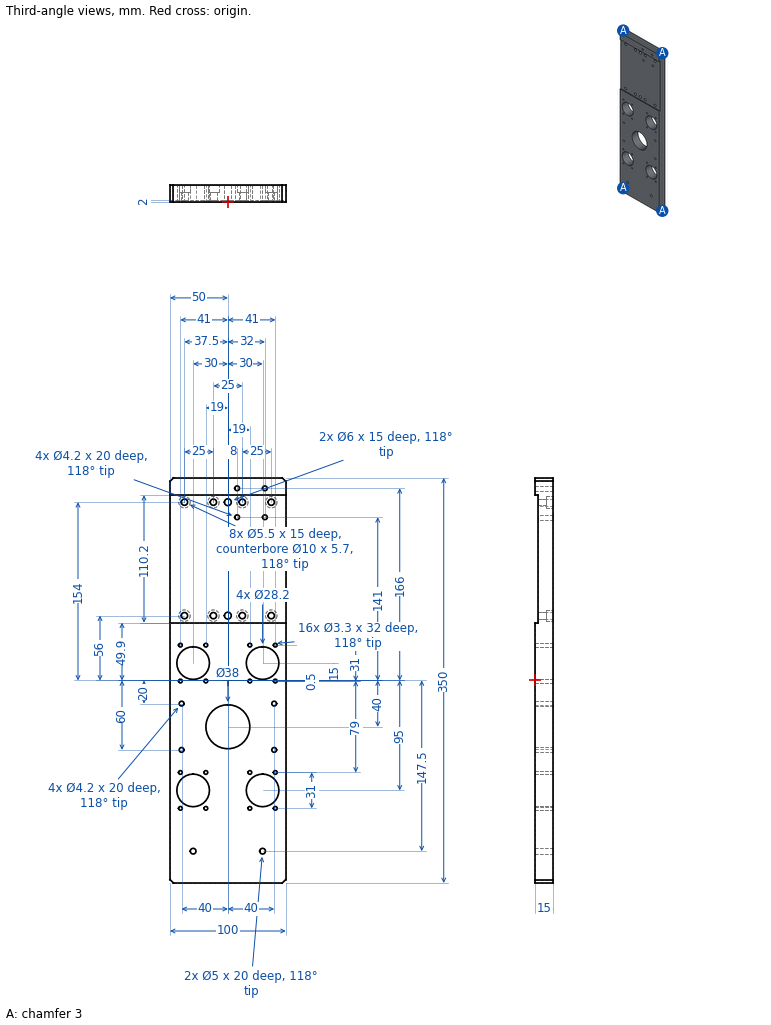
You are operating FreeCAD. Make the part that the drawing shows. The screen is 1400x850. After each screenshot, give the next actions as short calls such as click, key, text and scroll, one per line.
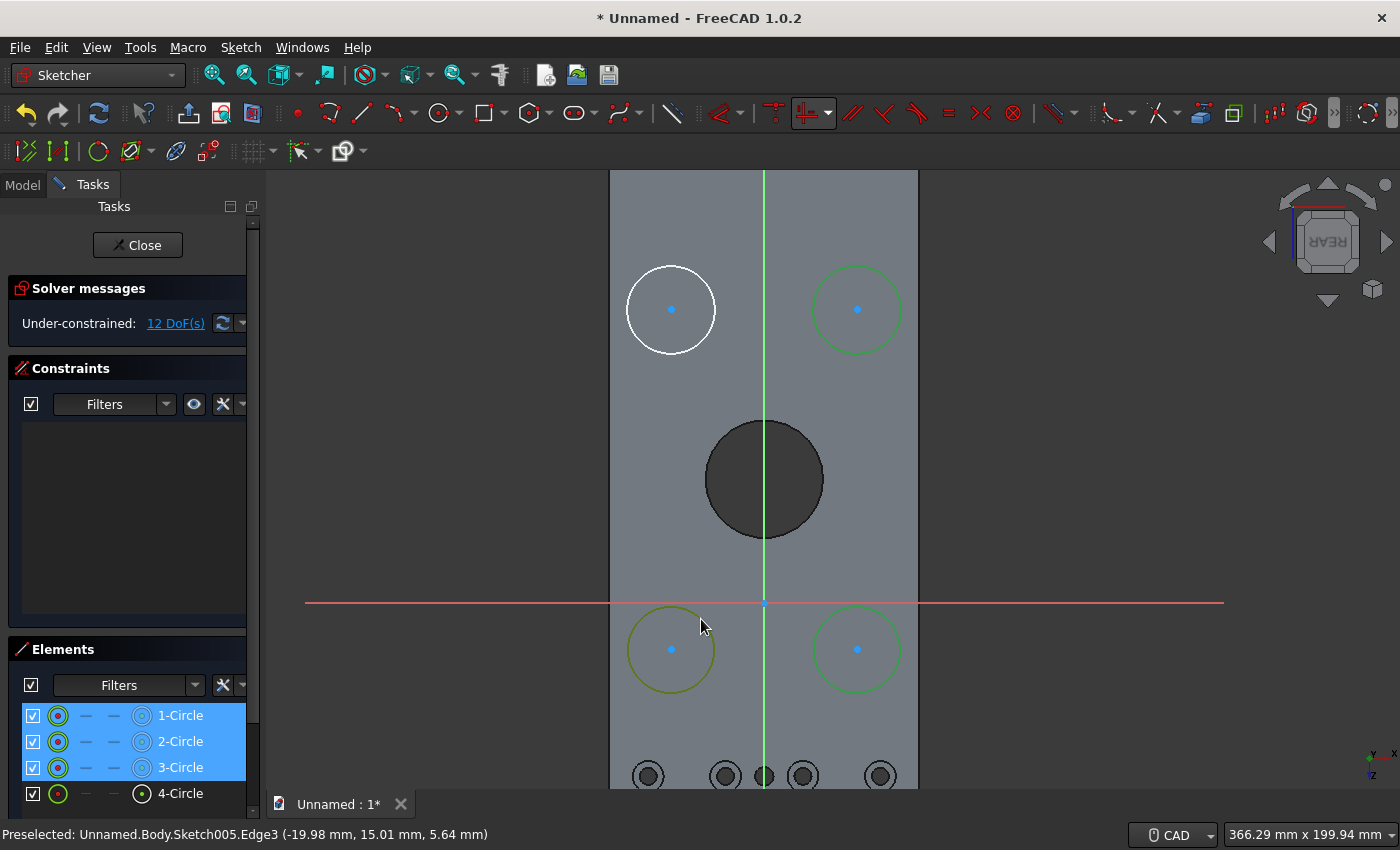
click(702, 279)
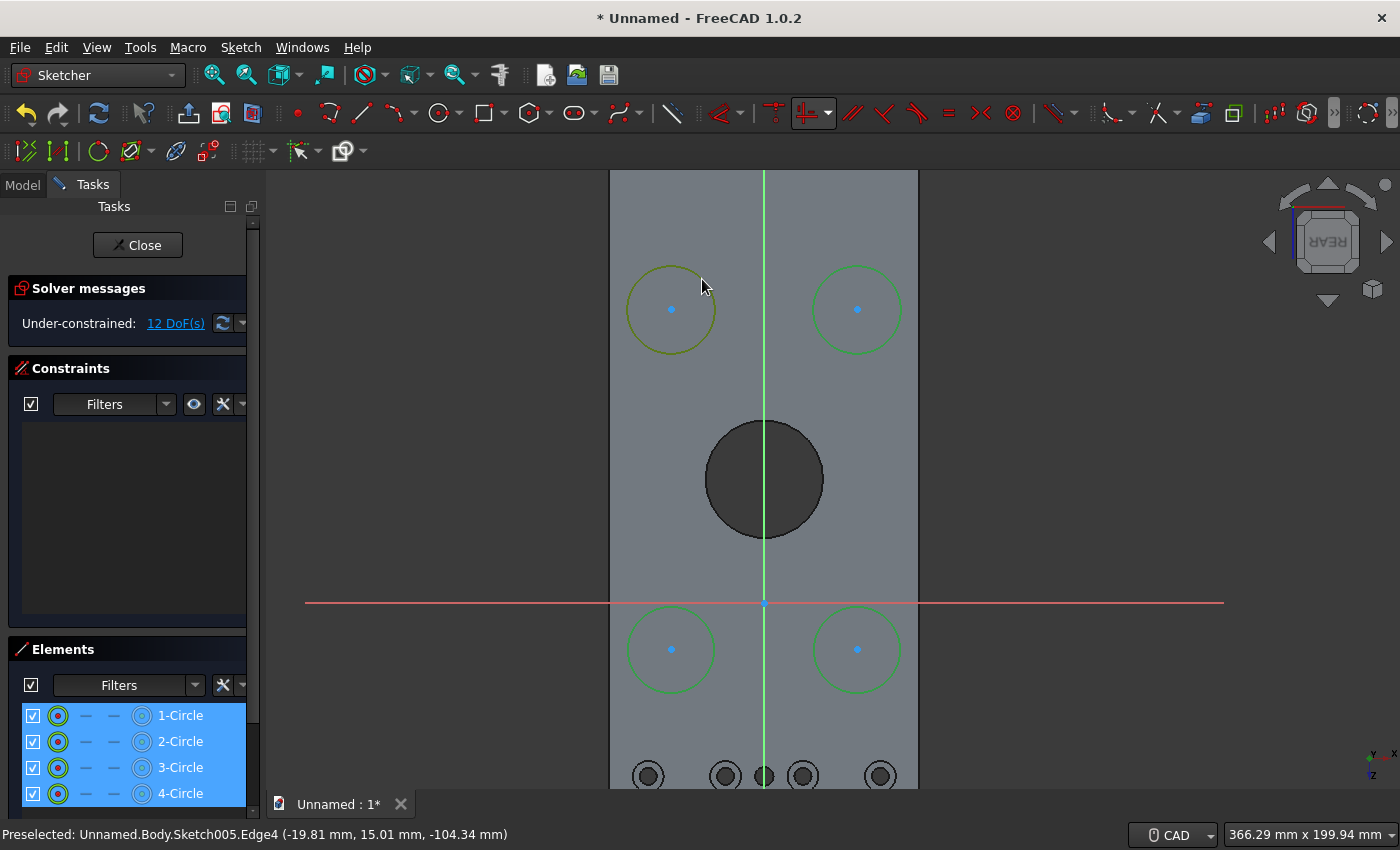
click(950, 114)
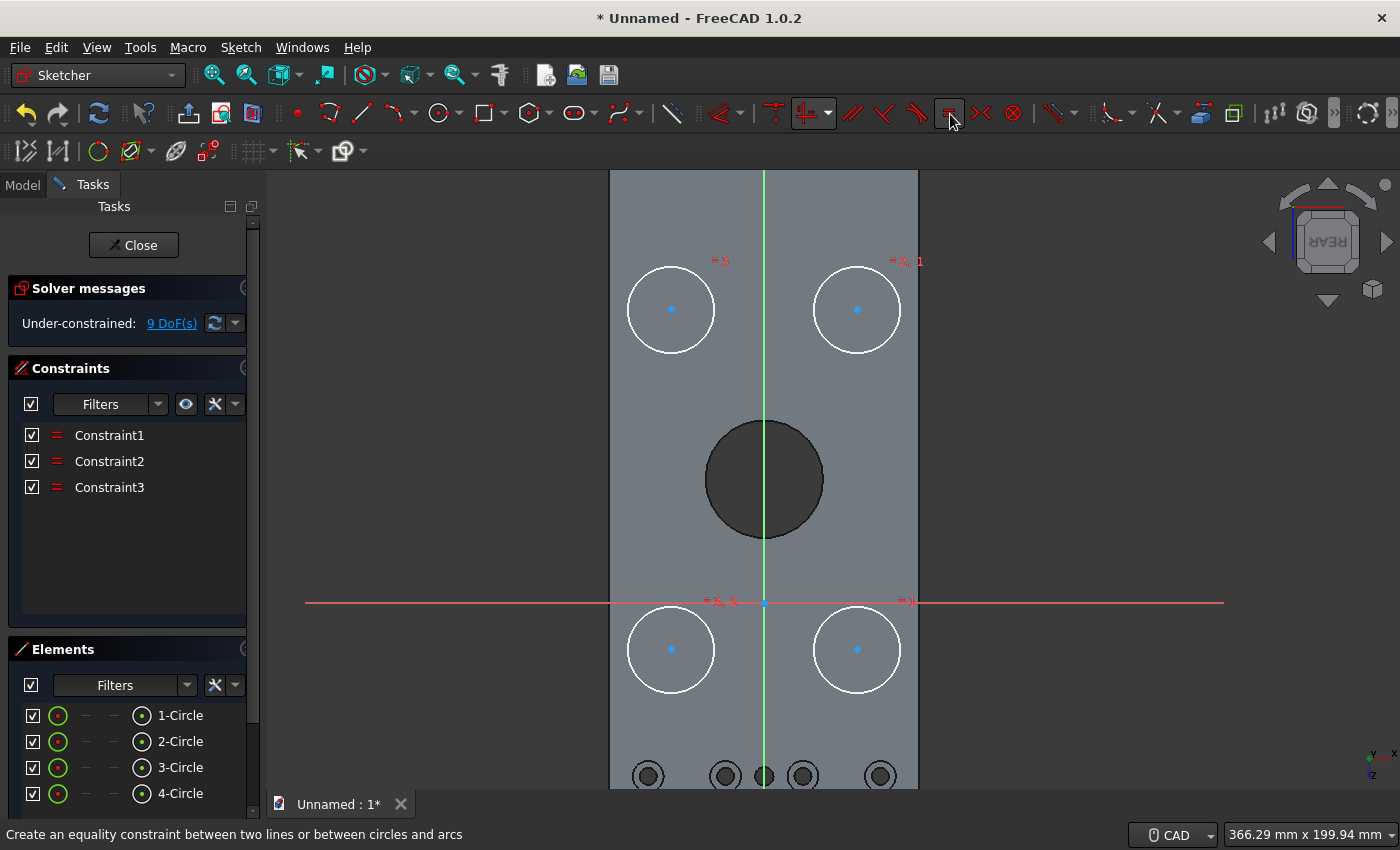
click(857, 650)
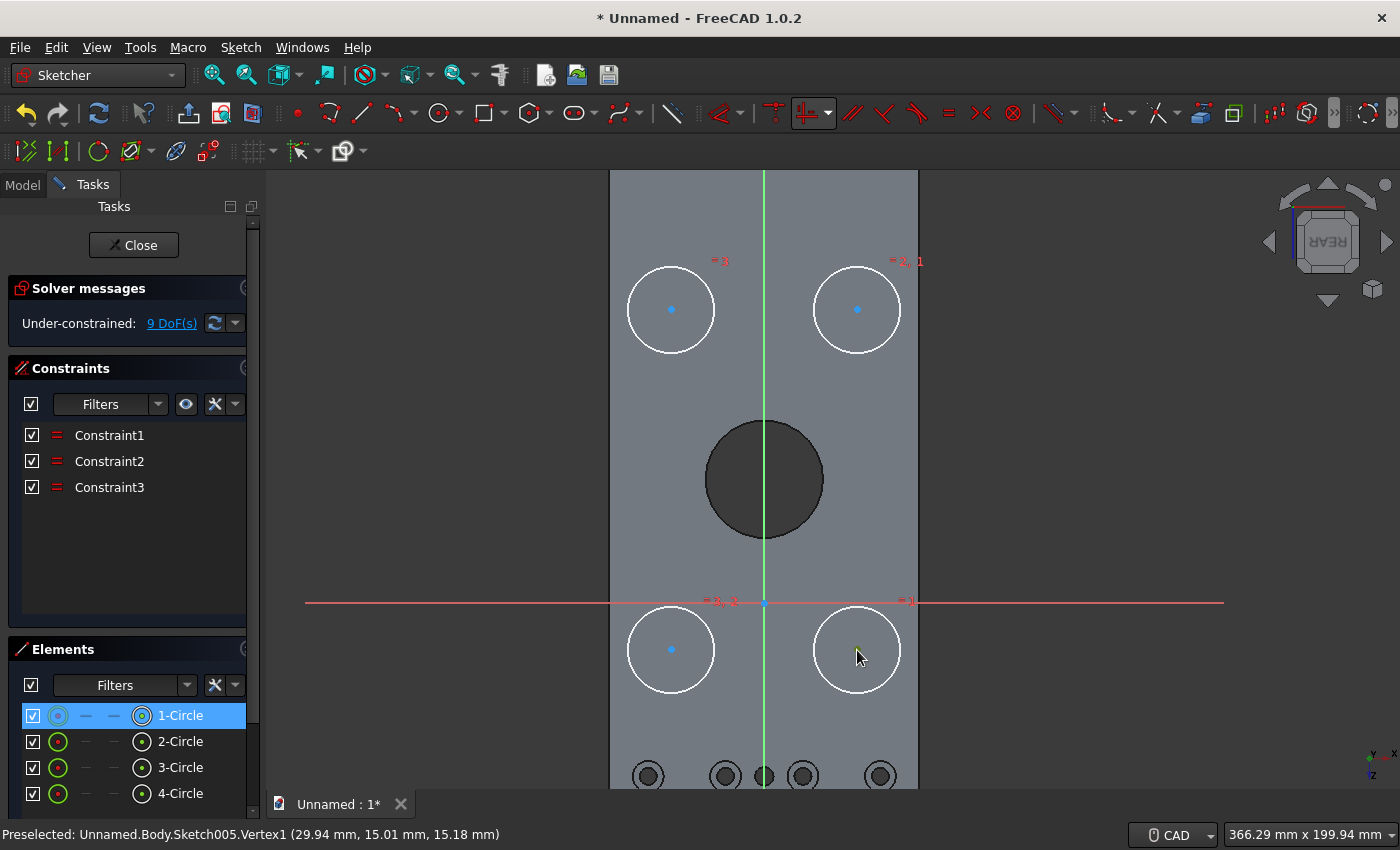
click(857, 310)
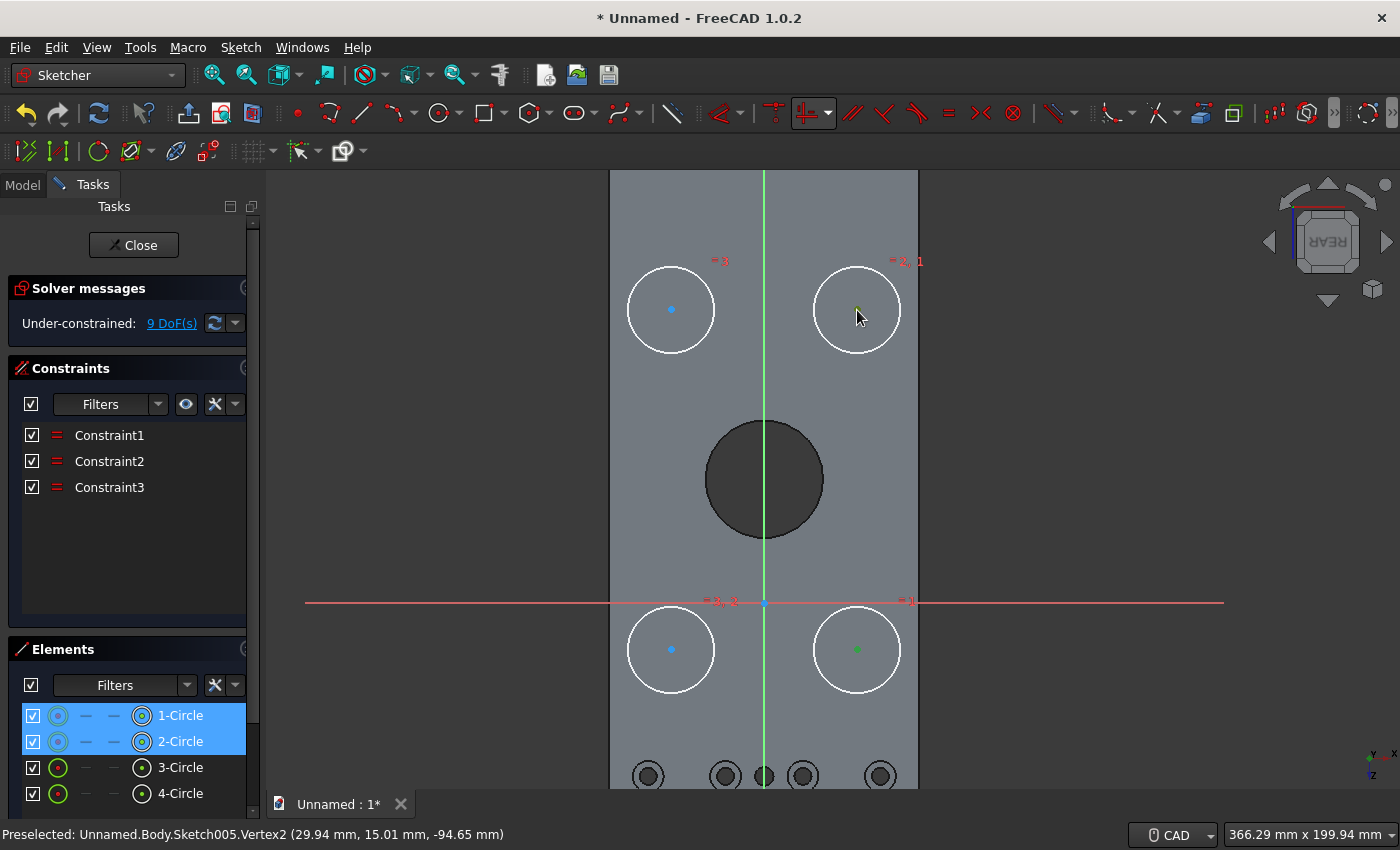
key(v)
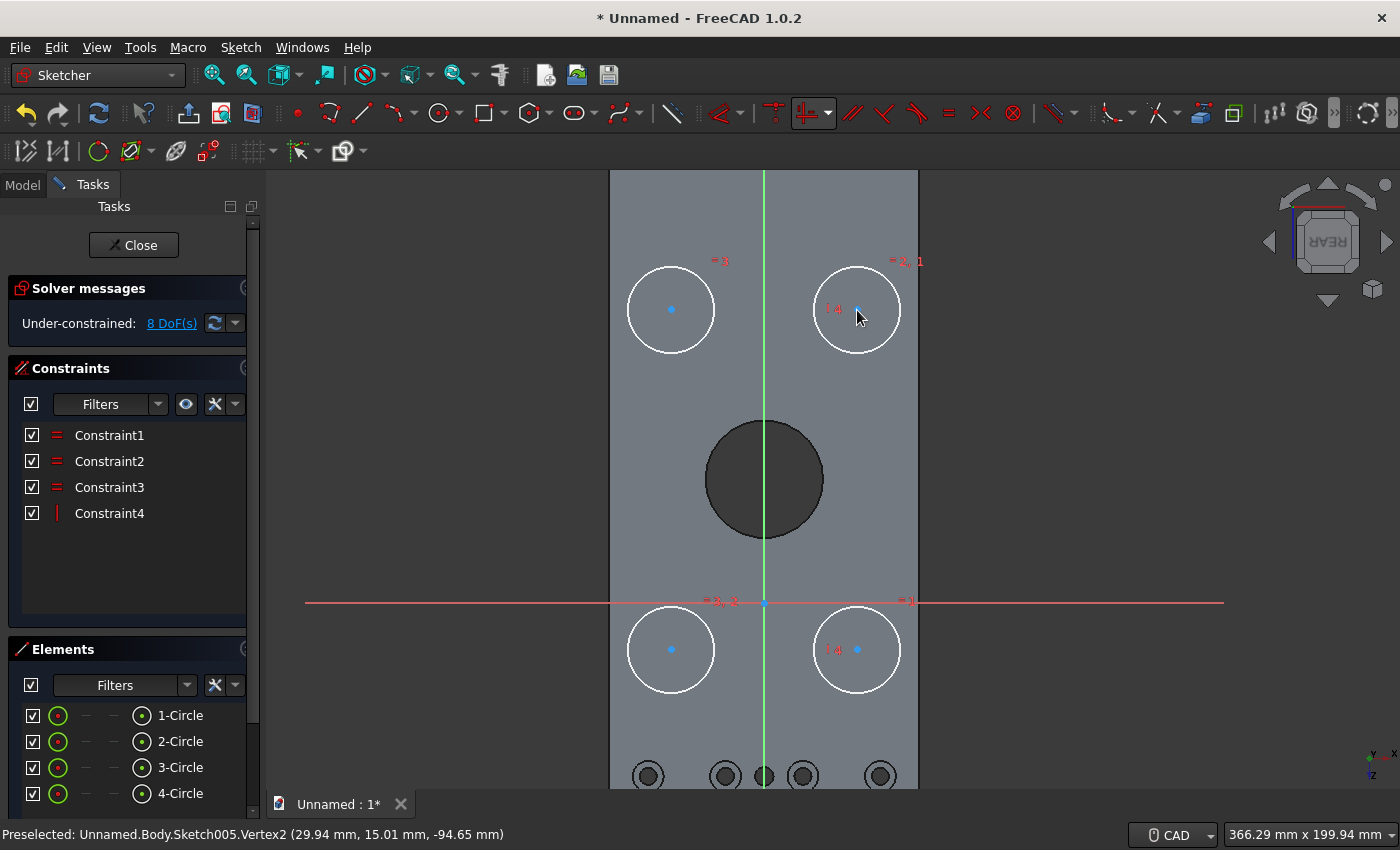
click(857, 650)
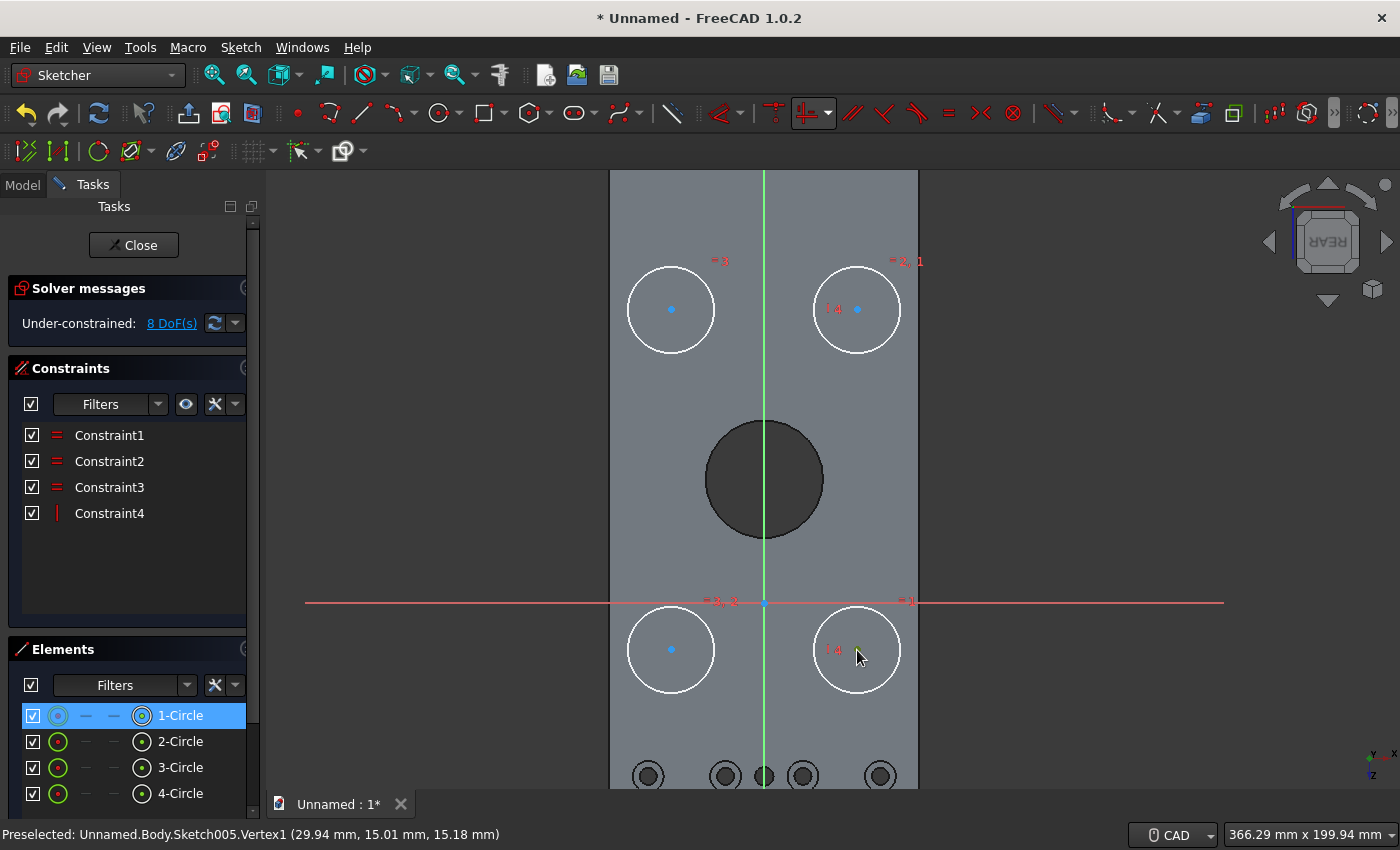
click(671, 650)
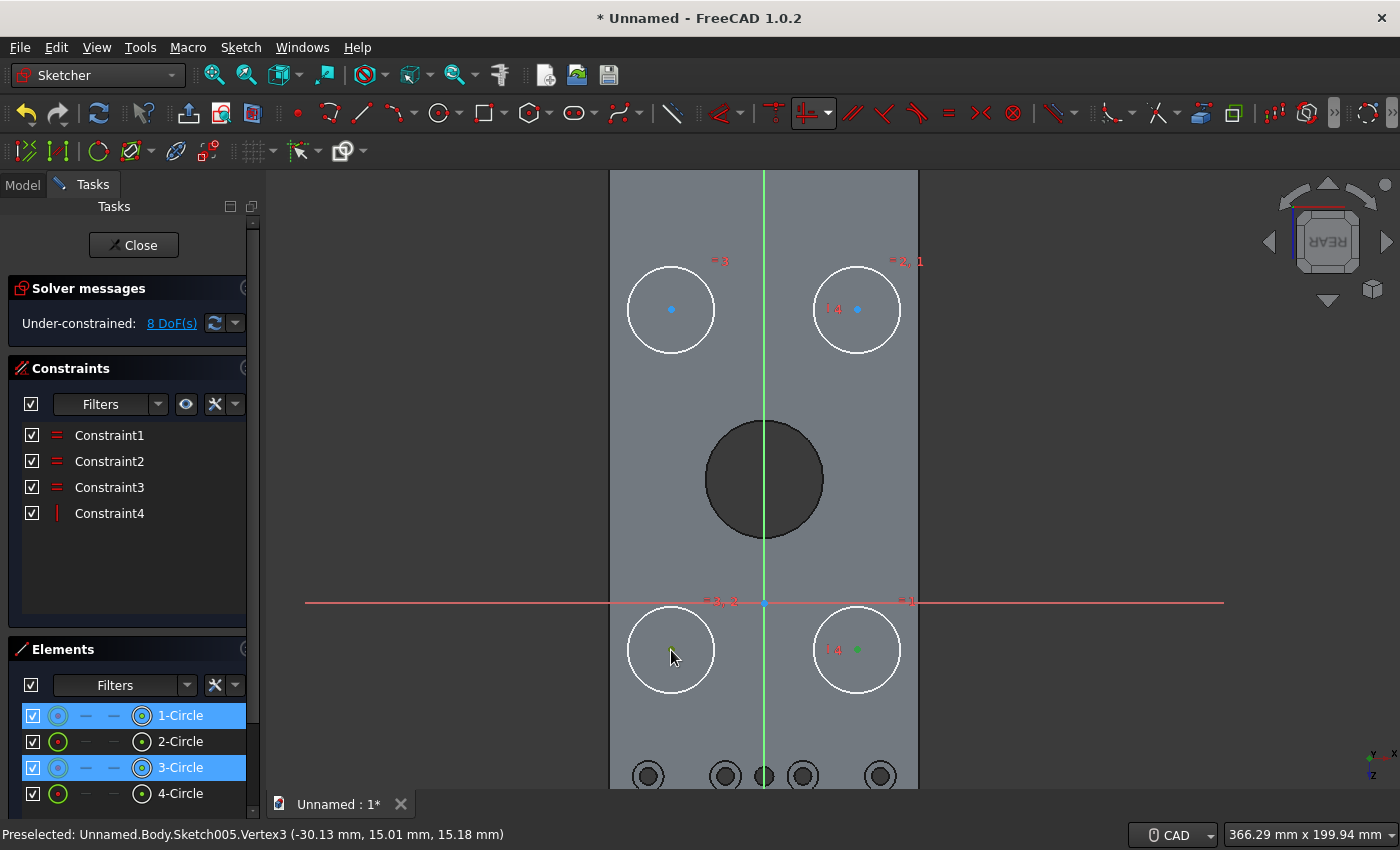
key(h)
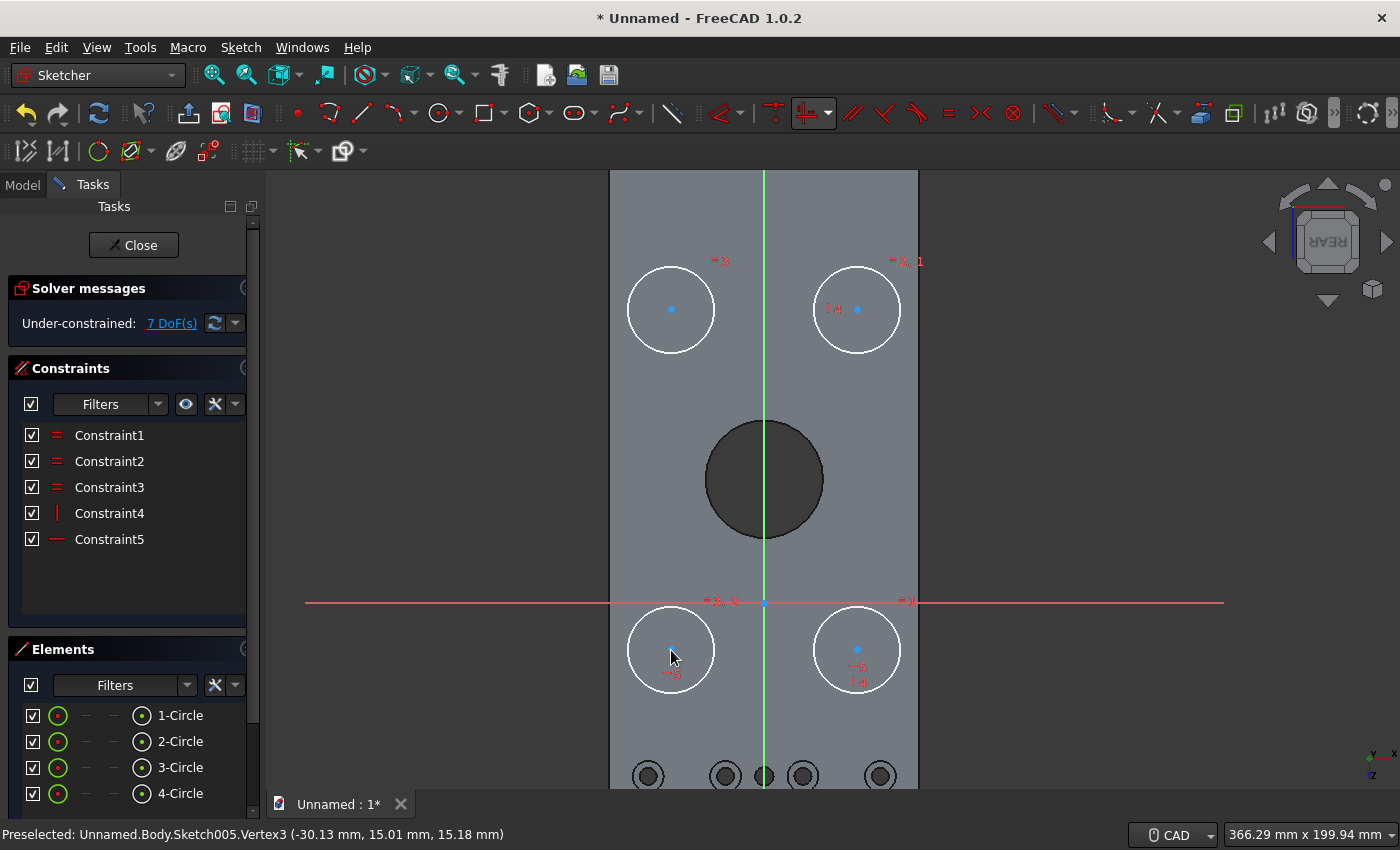
click(671, 650)